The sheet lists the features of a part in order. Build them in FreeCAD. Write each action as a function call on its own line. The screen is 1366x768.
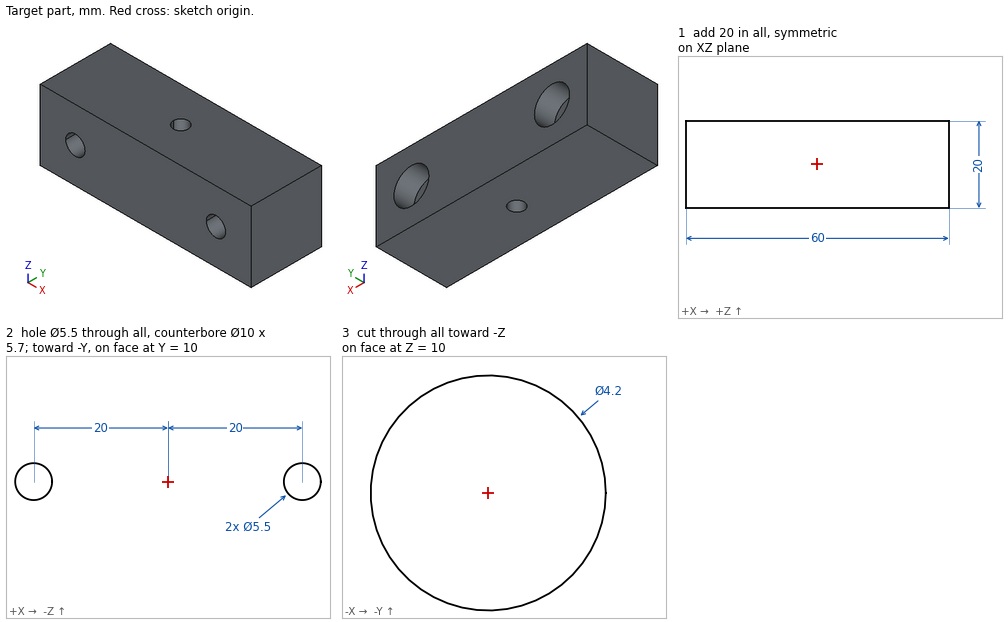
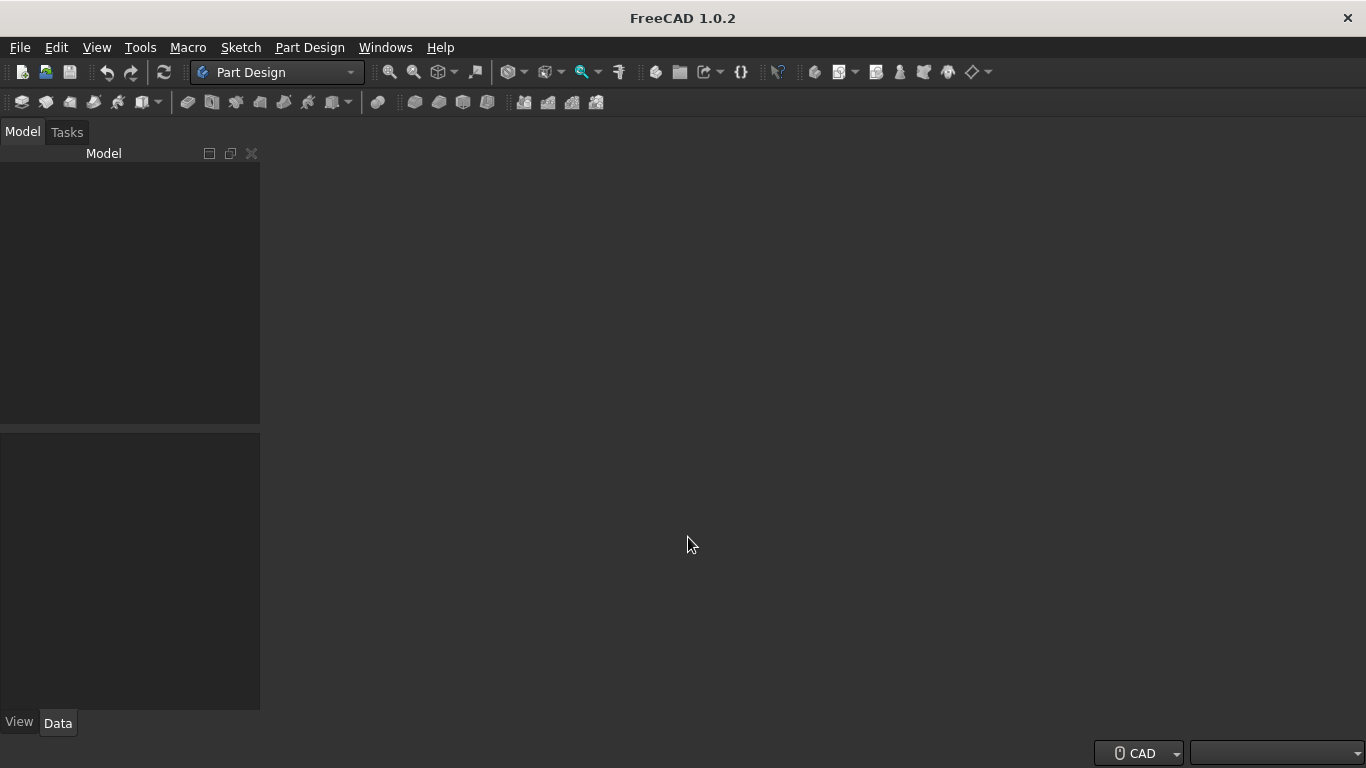
key(ctrl+n)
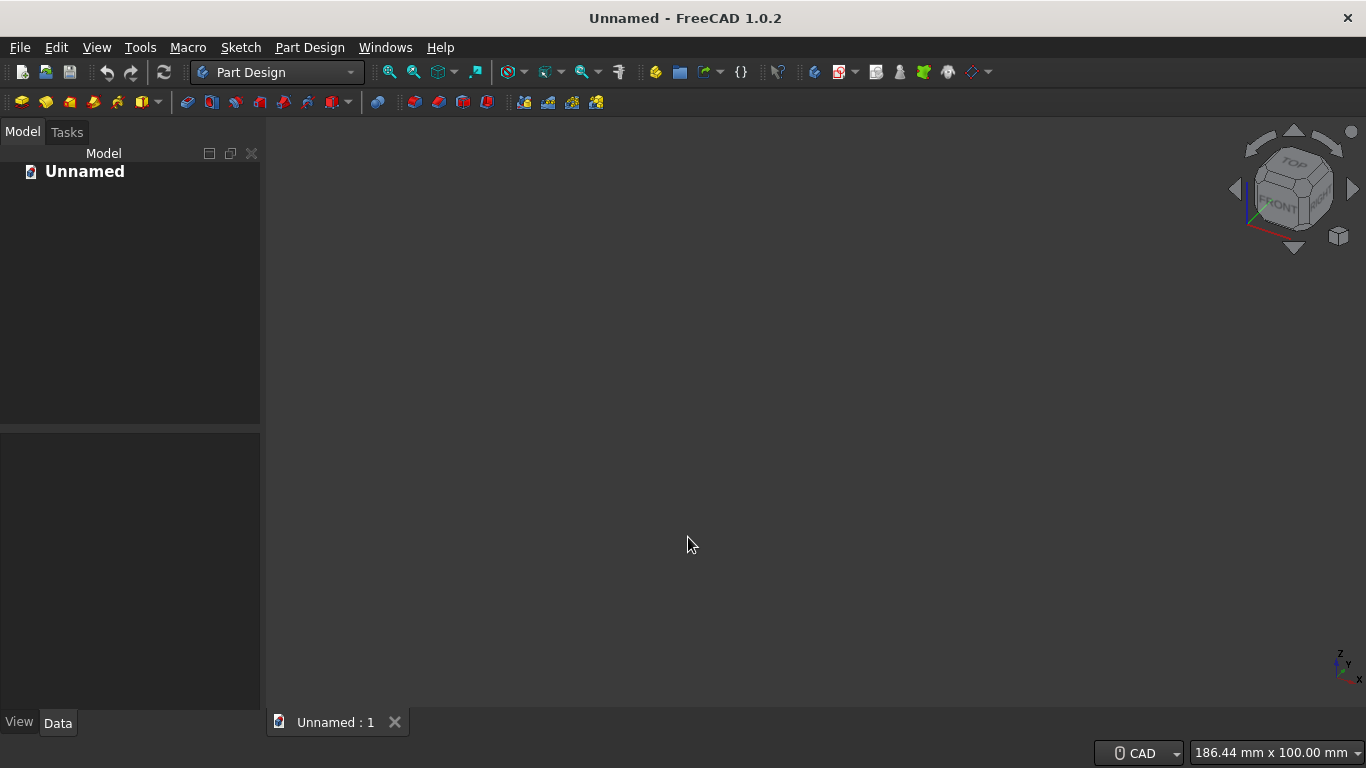
click(840, 72)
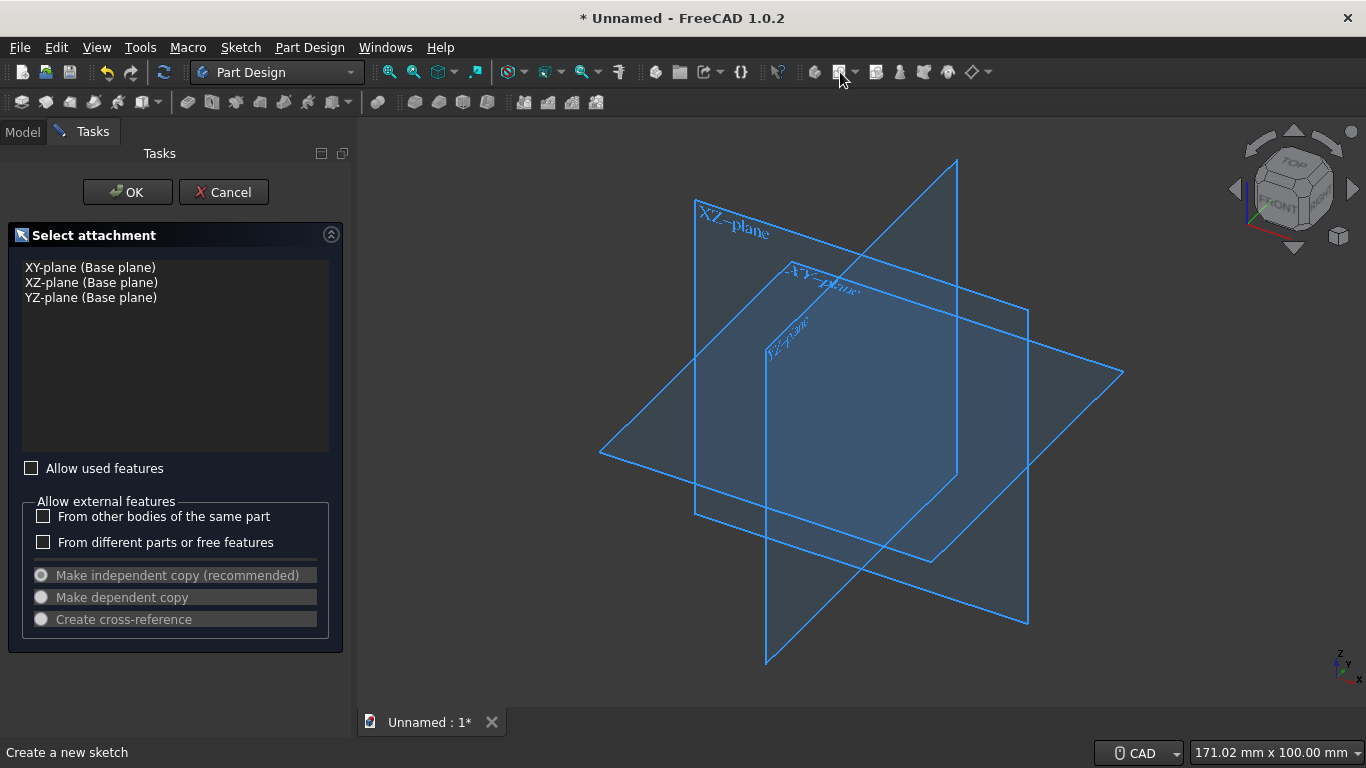
click(82, 282)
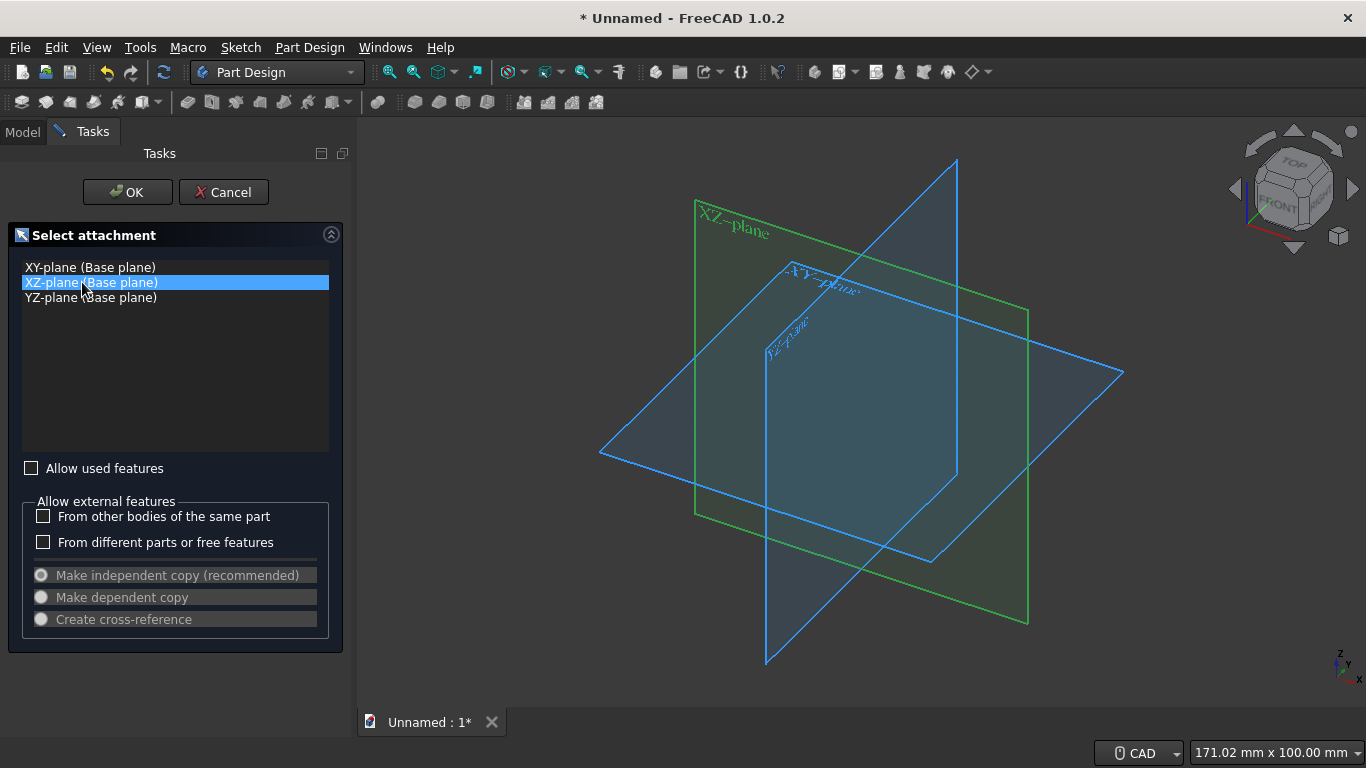
click(128, 192)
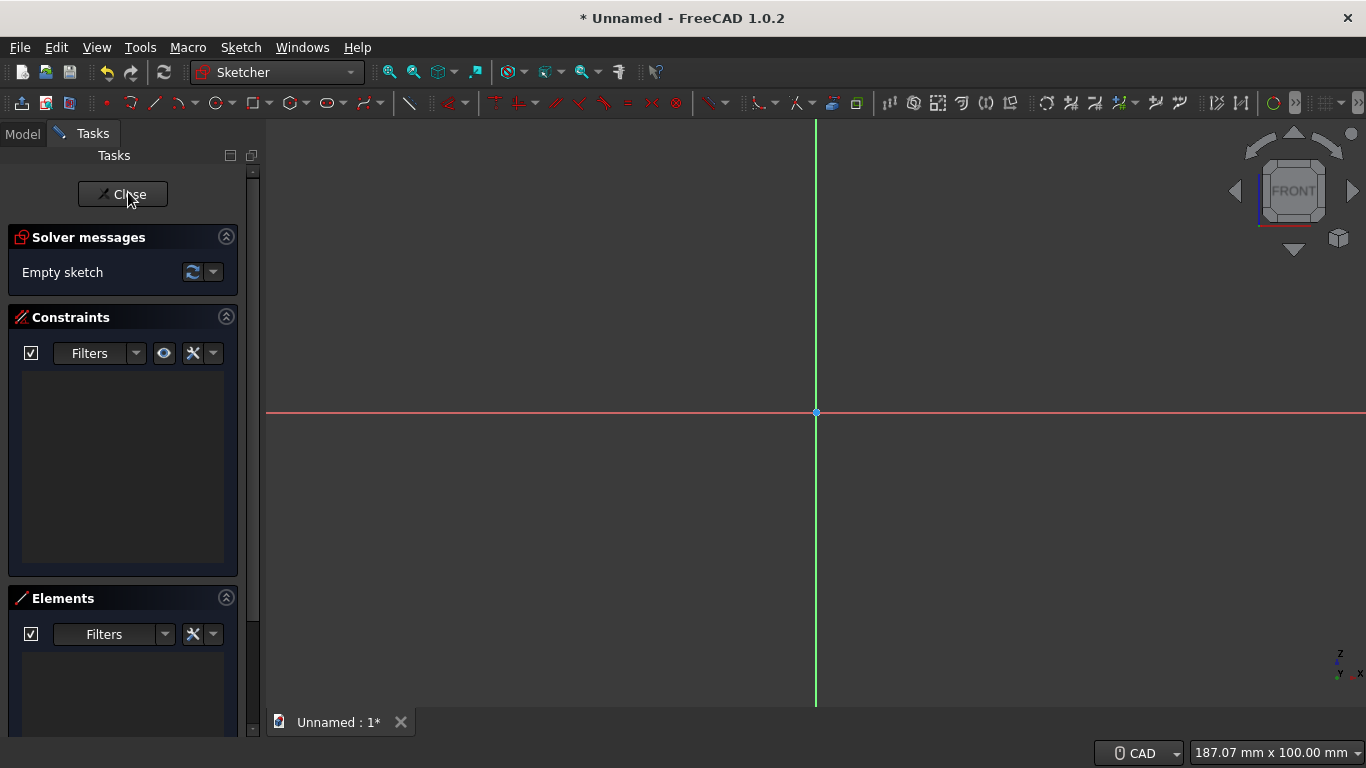
scroll(899, 413, up, 3)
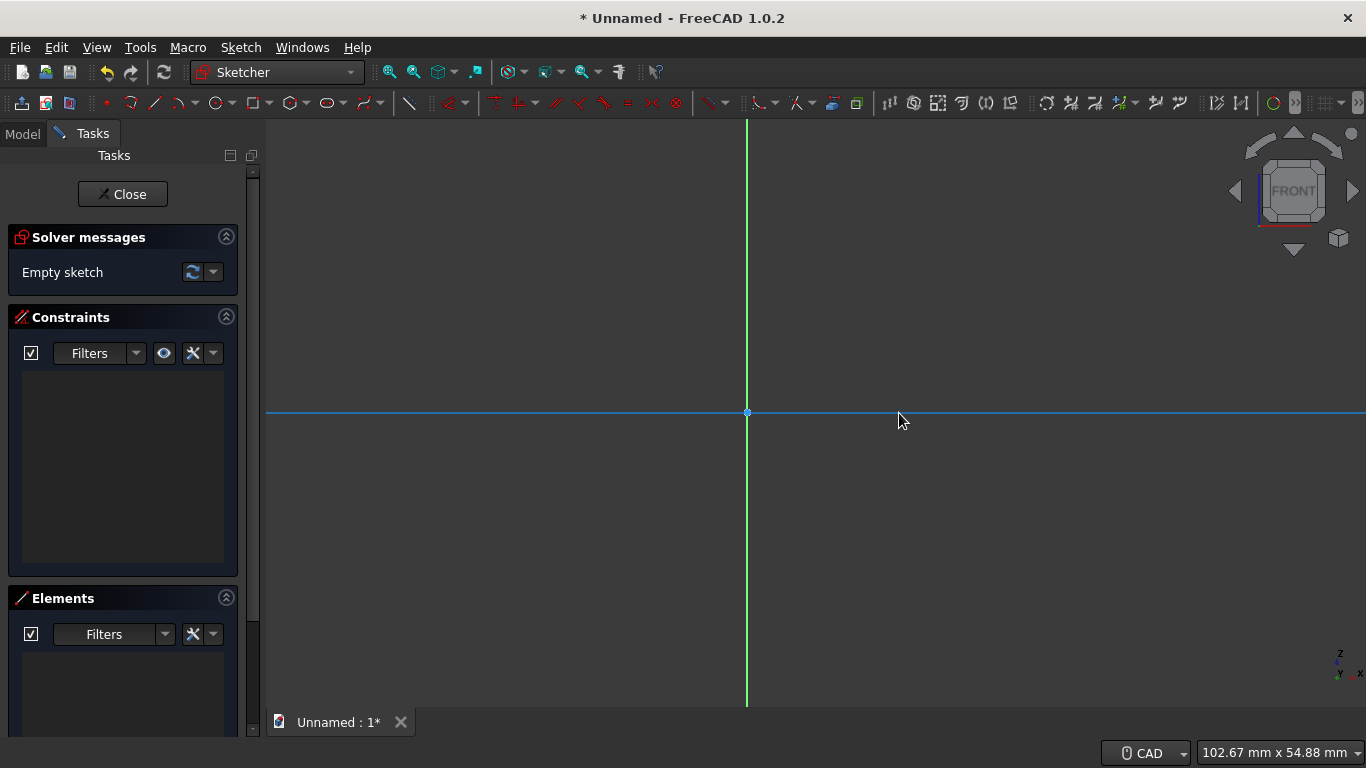
click(272, 104)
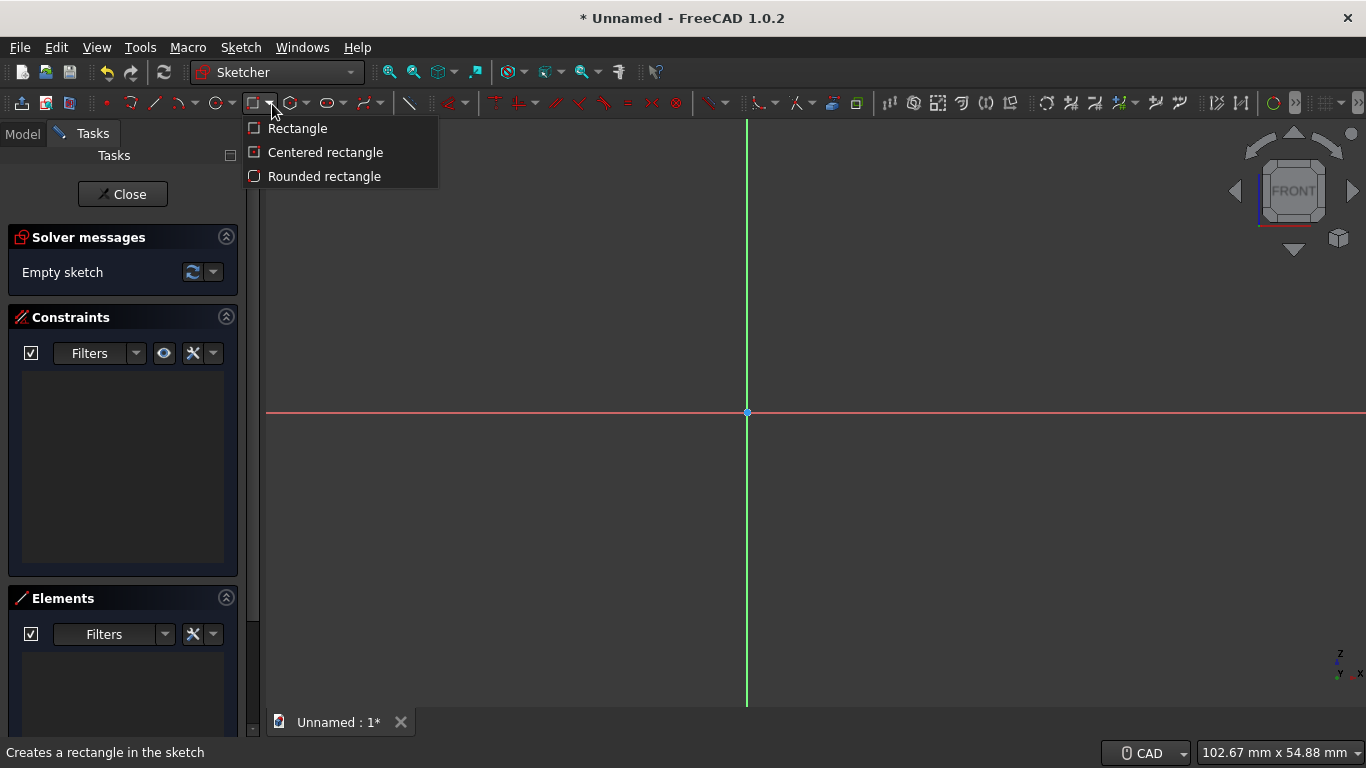
click(340, 152)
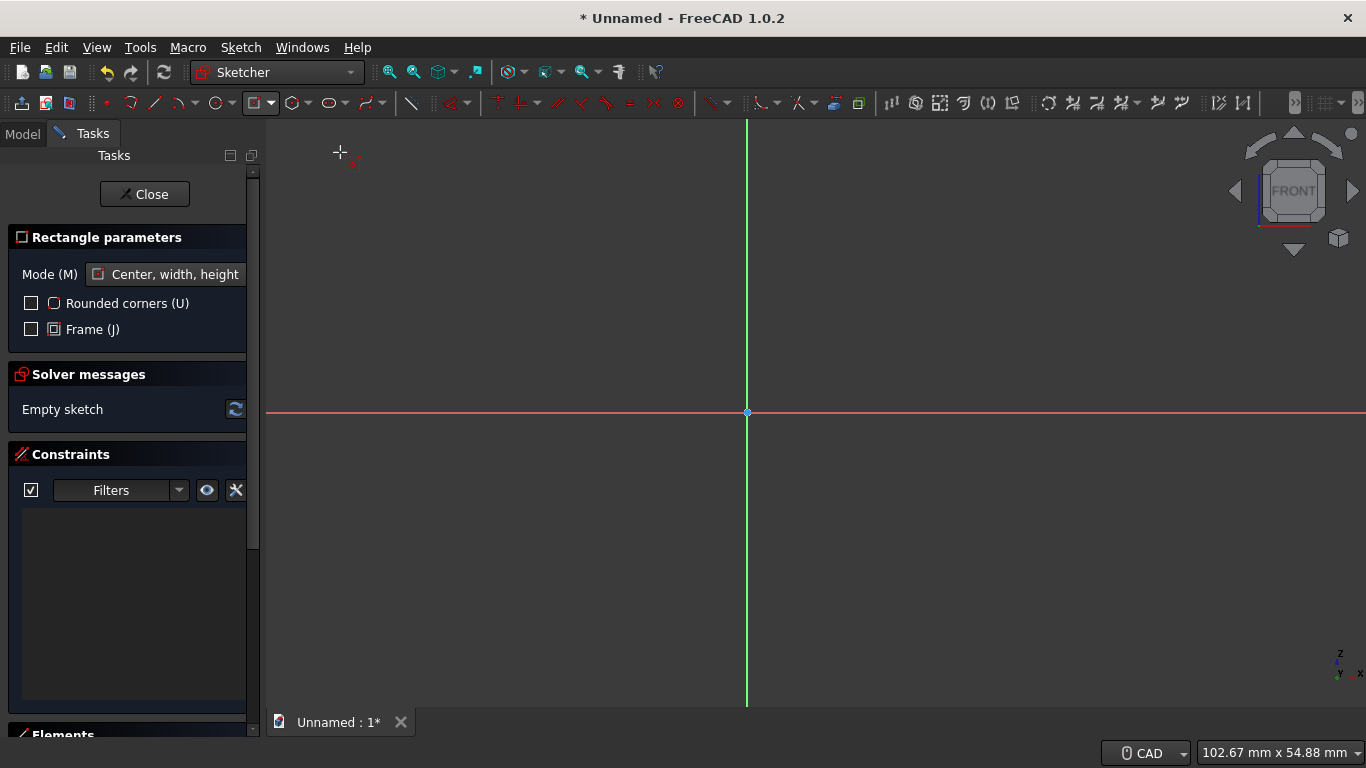
click(747, 413)
move(1069, 305)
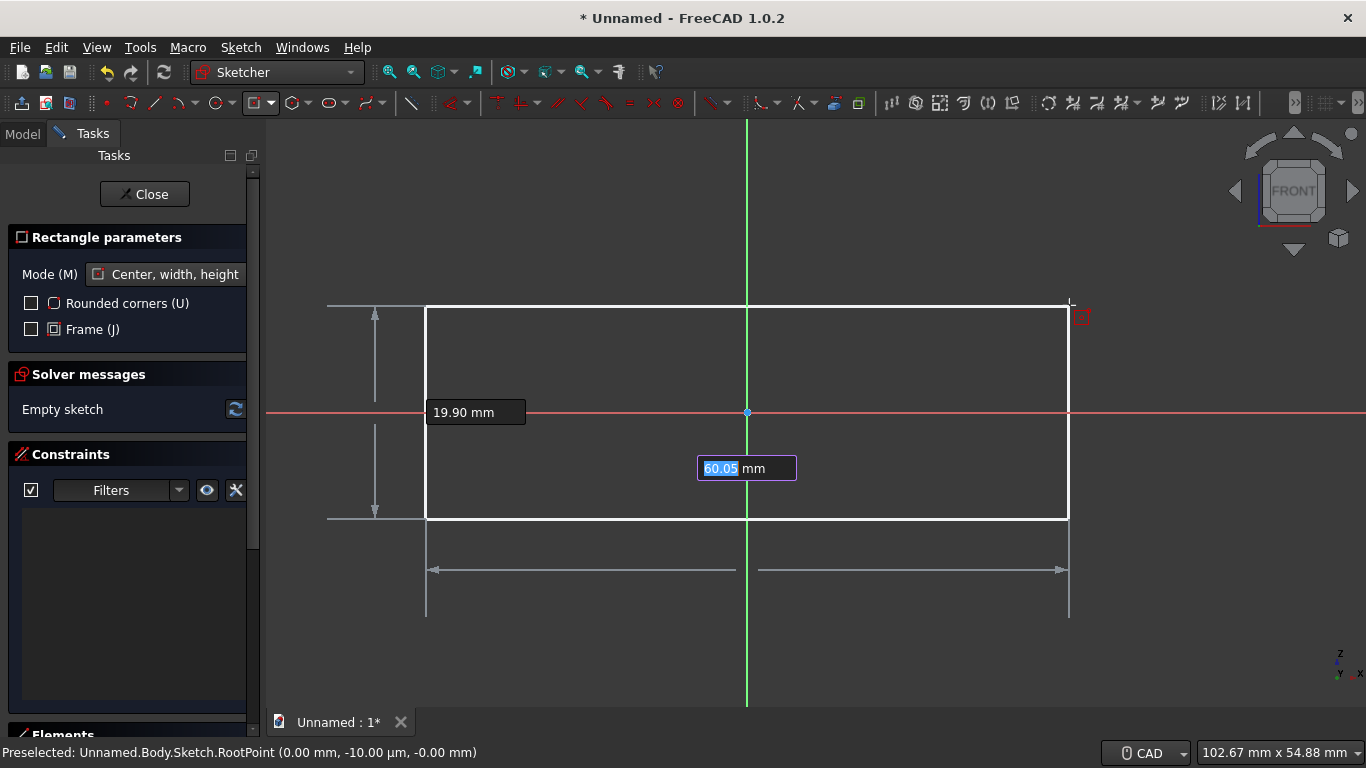
text(60)
key(Tab)
text(20)
key(Return)
key(Escape)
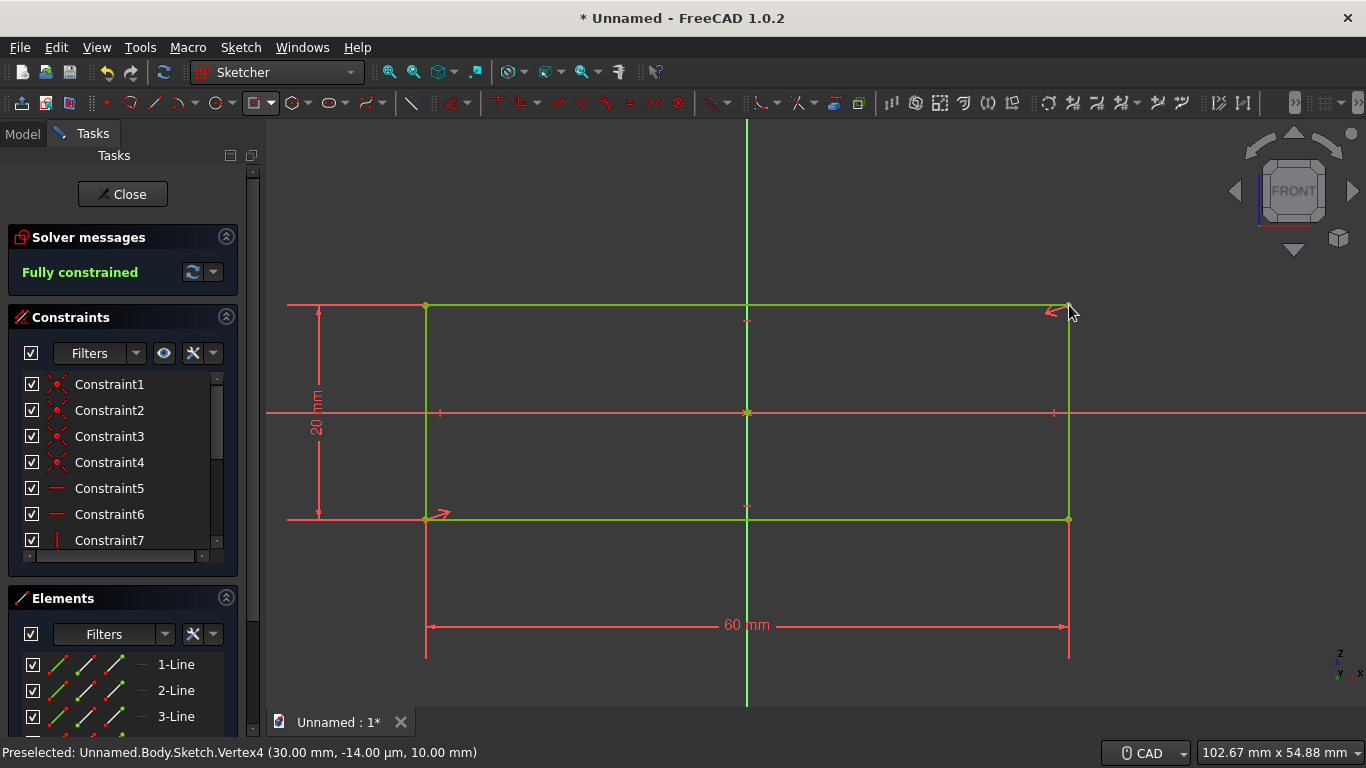
click(123, 194)